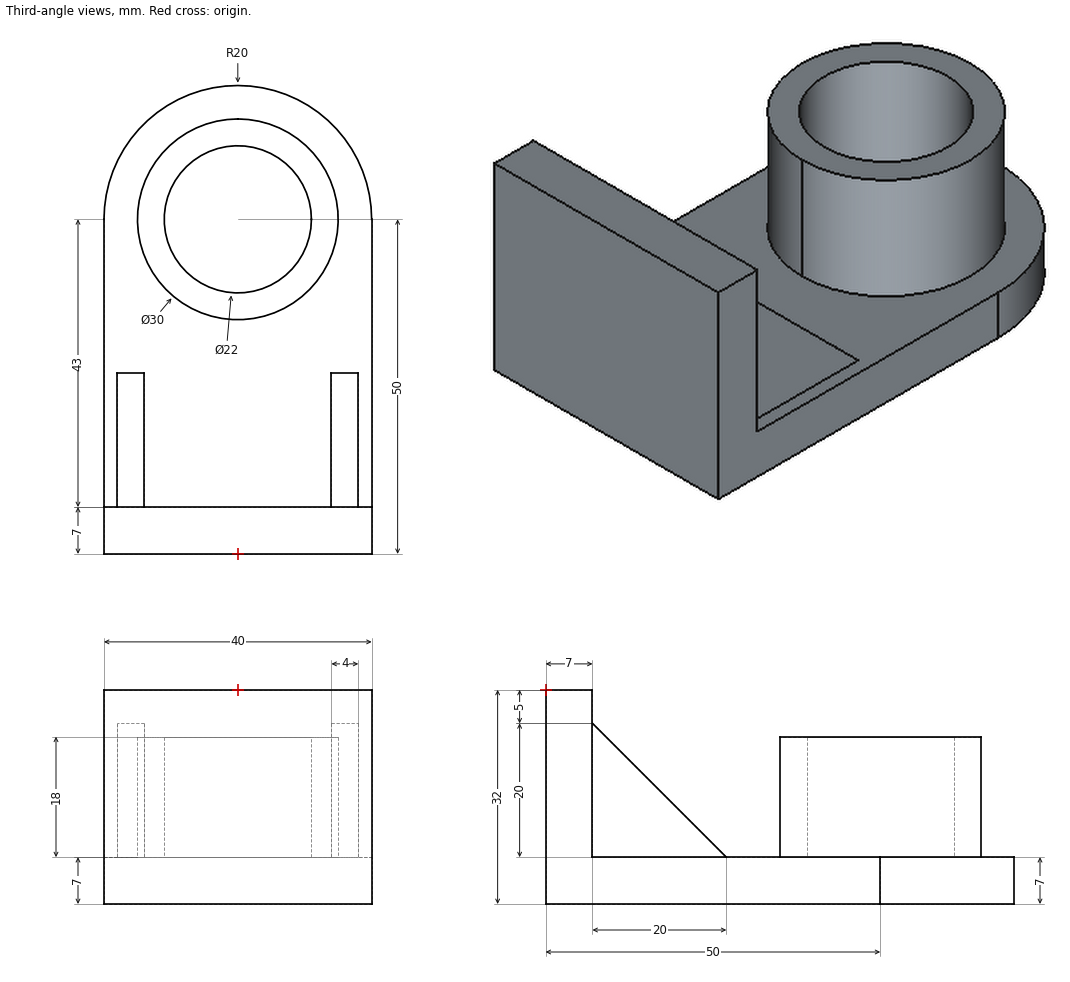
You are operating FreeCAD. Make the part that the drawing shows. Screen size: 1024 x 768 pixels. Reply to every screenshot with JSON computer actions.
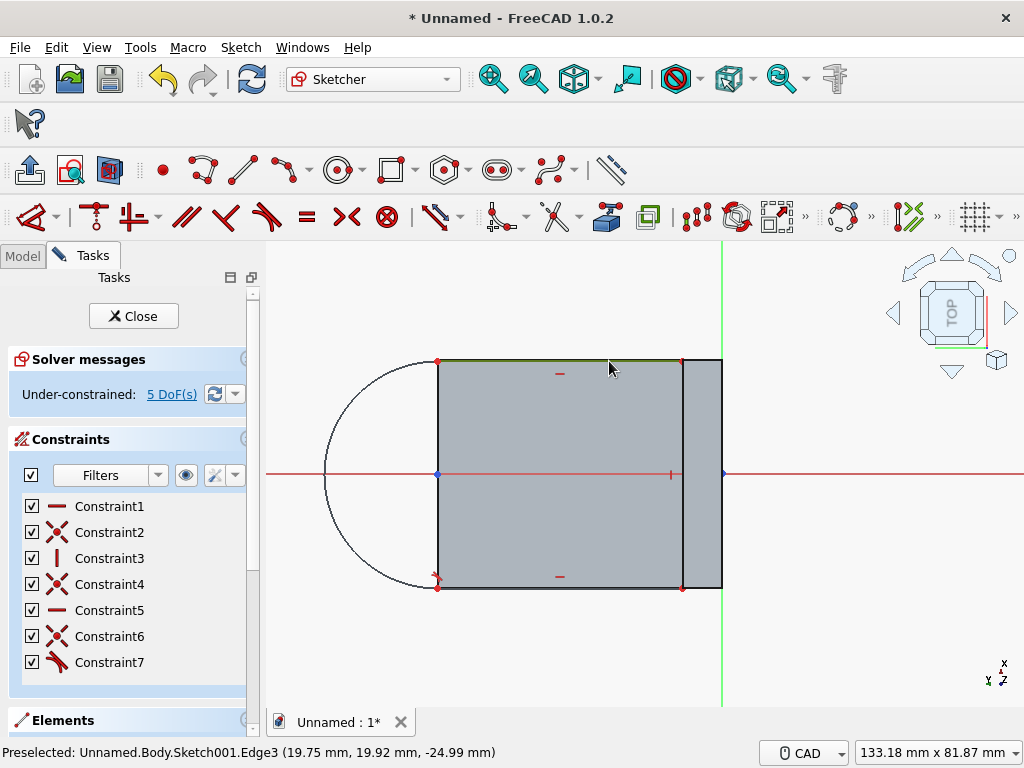
{"action": "left_click", "coordinate": [346, 408]}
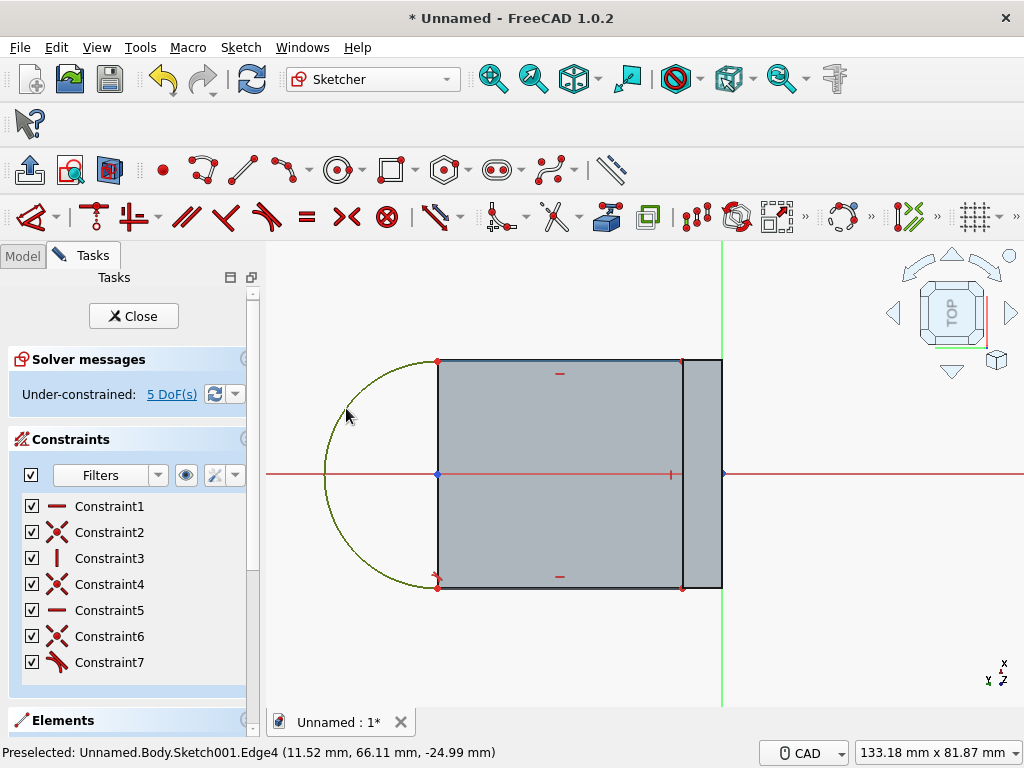
{"action": "left_click", "coordinate": [268, 218]}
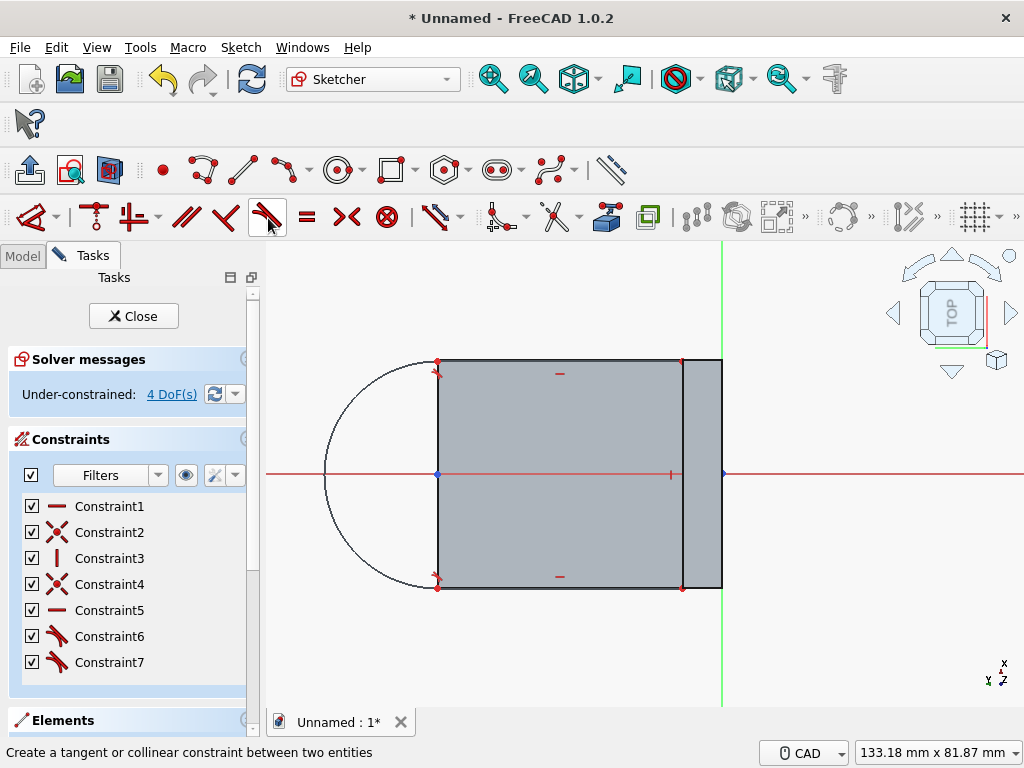
{"action": "left_click", "coordinate": [438, 475]}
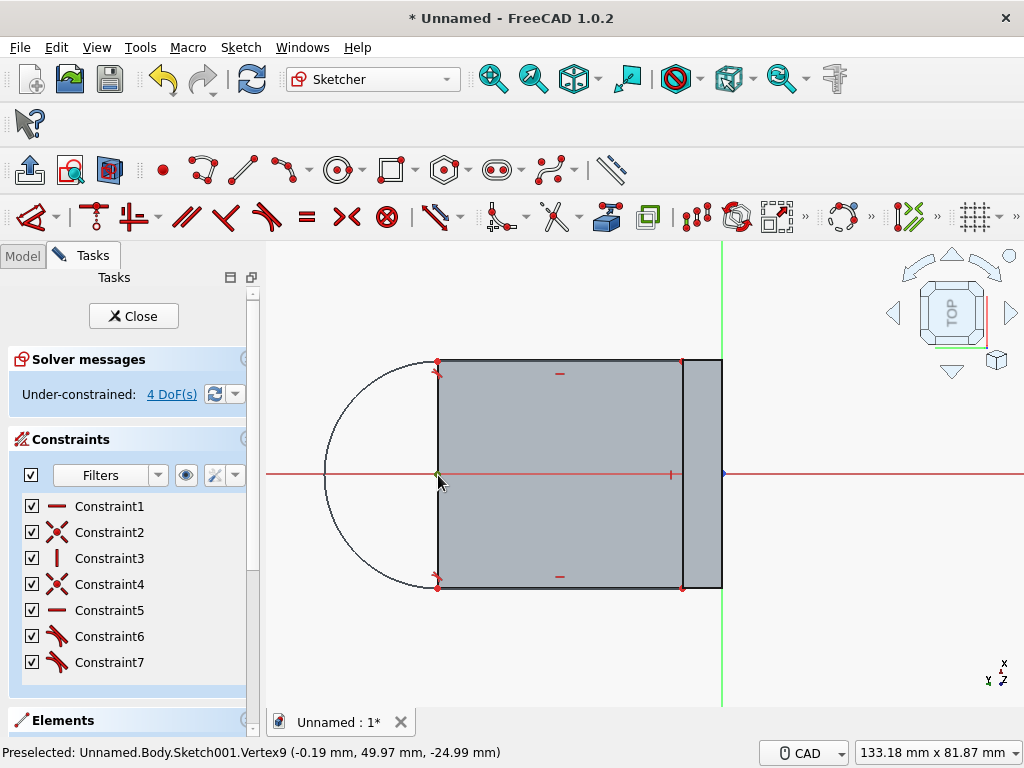
{"action": "left_click", "coordinate": [375, 474]}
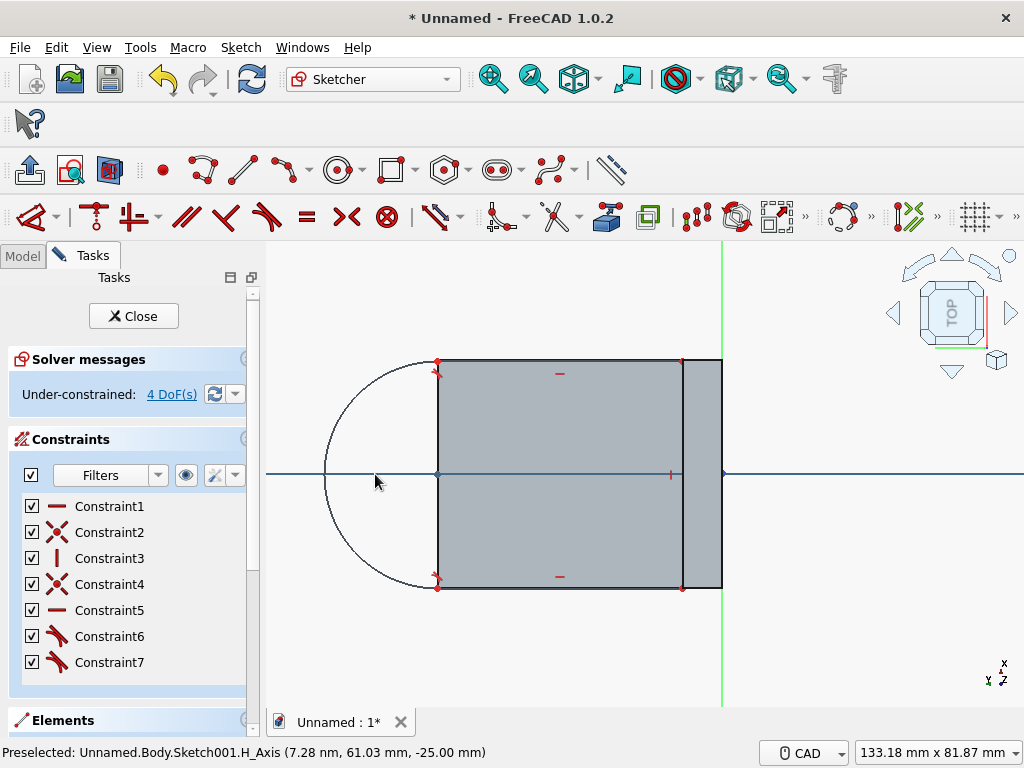
{"action": "left_click", "coordinate": [94, 218]}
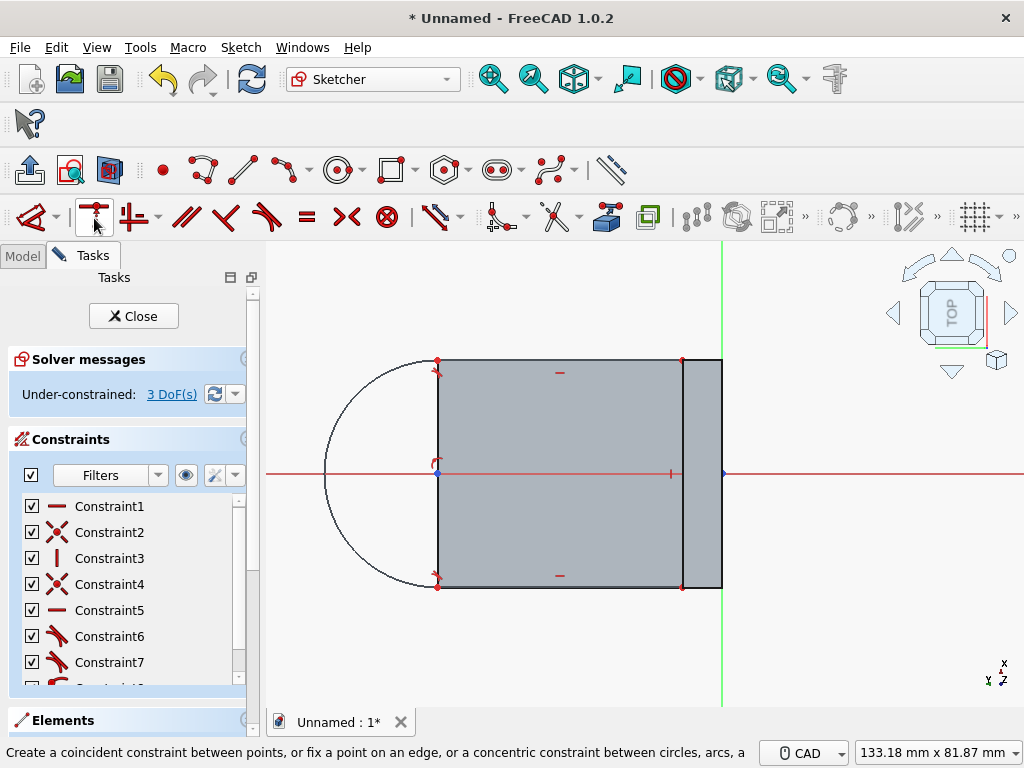
{"action": "left_click", "coordinate": [32, 218]}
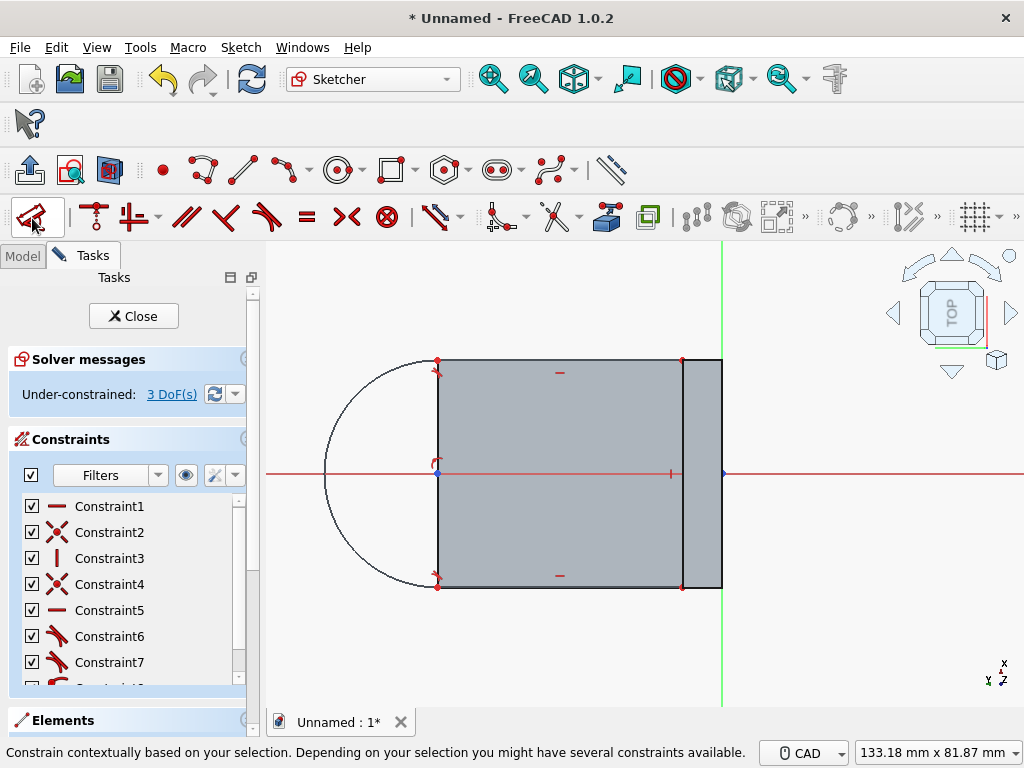
{"action": "left_click", "coordinate": [346, 407]}
{"action": "left_click", "coordinate": [320, 388]}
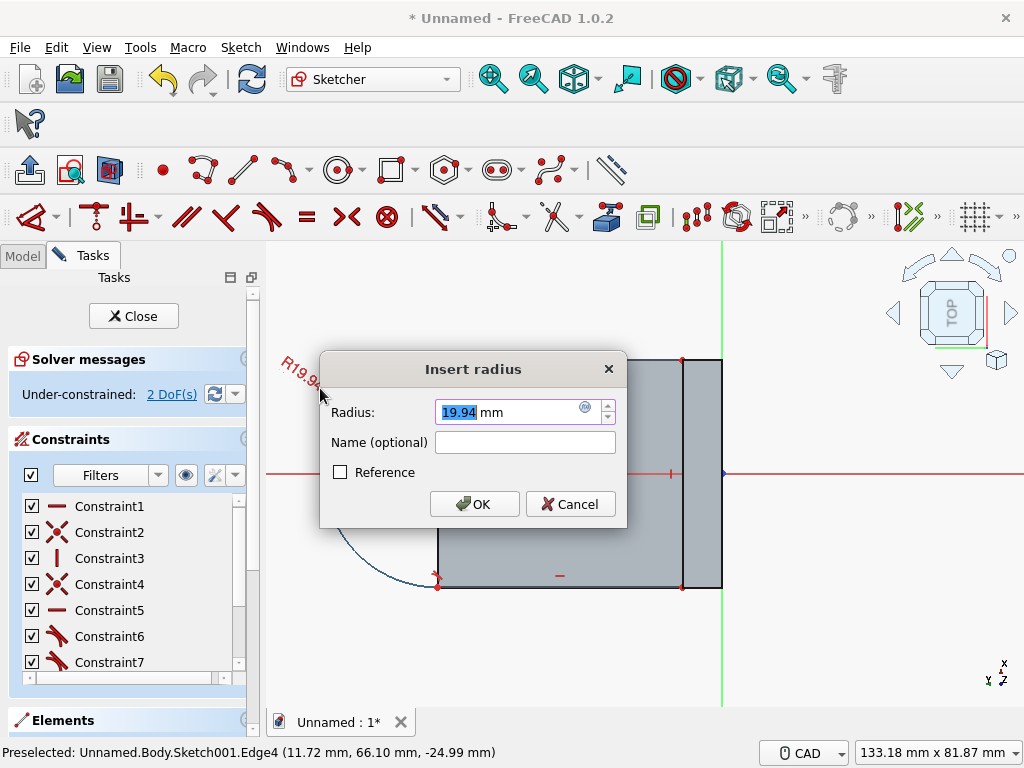
{"action": "type", "text": "20"}
{"action": "key", "text": "Return"}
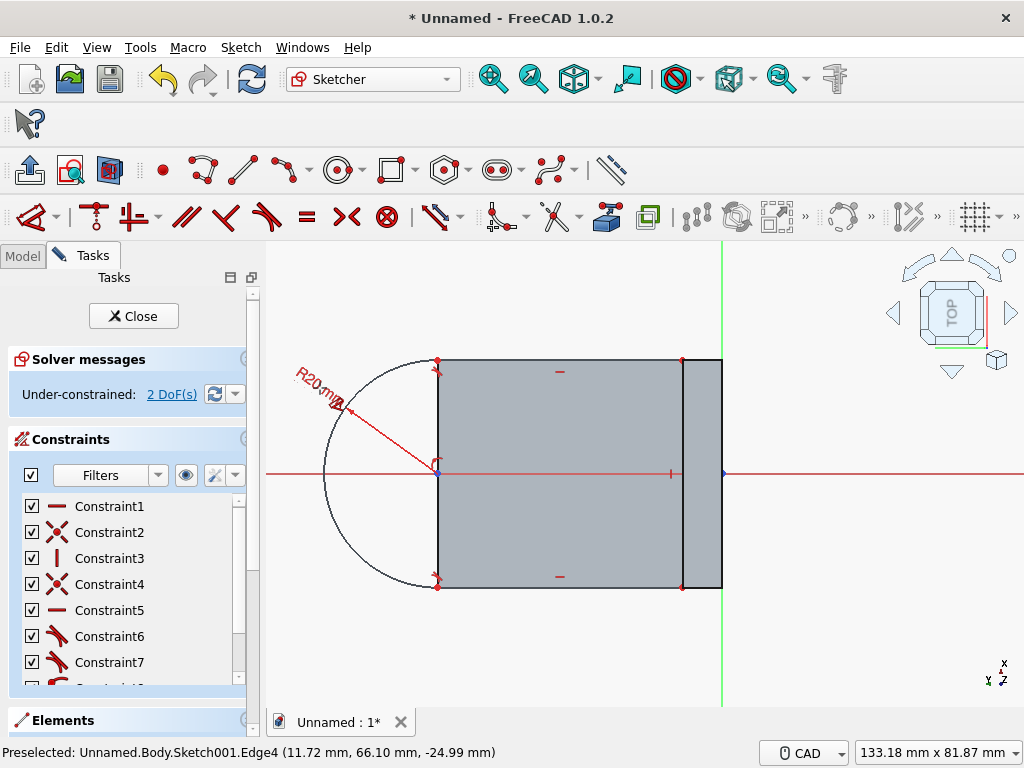
{"action": "left_click", "coordinate": [511, 588]}
{"action": "left_click", "coordinate": [560, 622]}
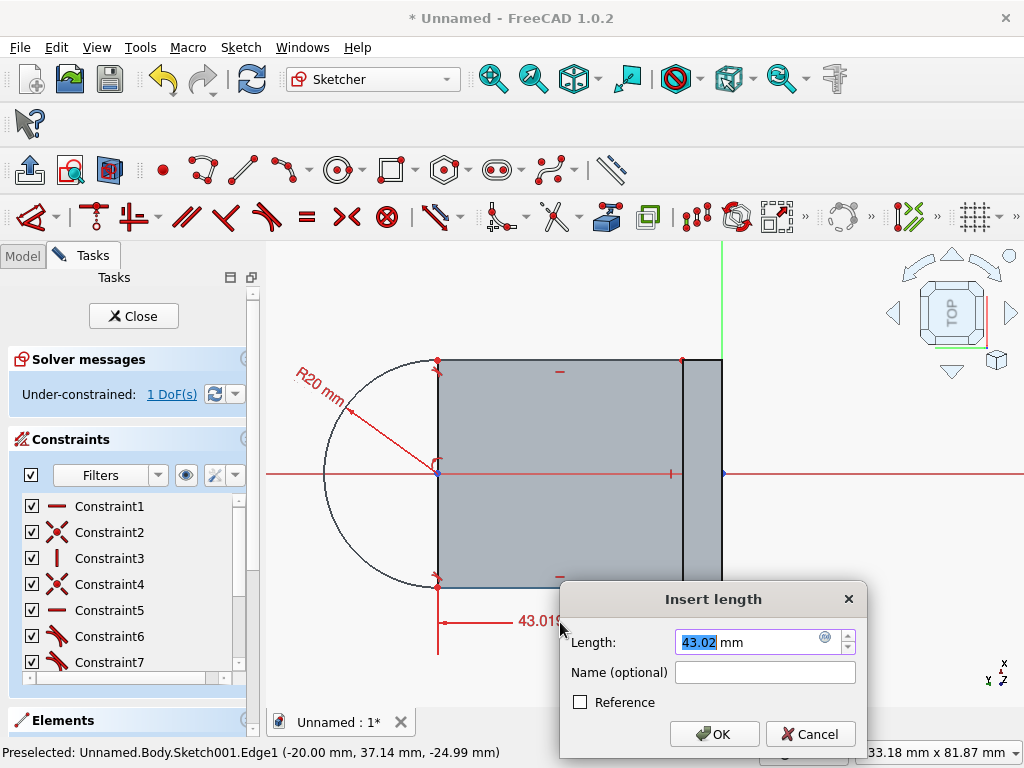
{"action": "type", "text": "43"}
{"action": "key", "text": "Return"}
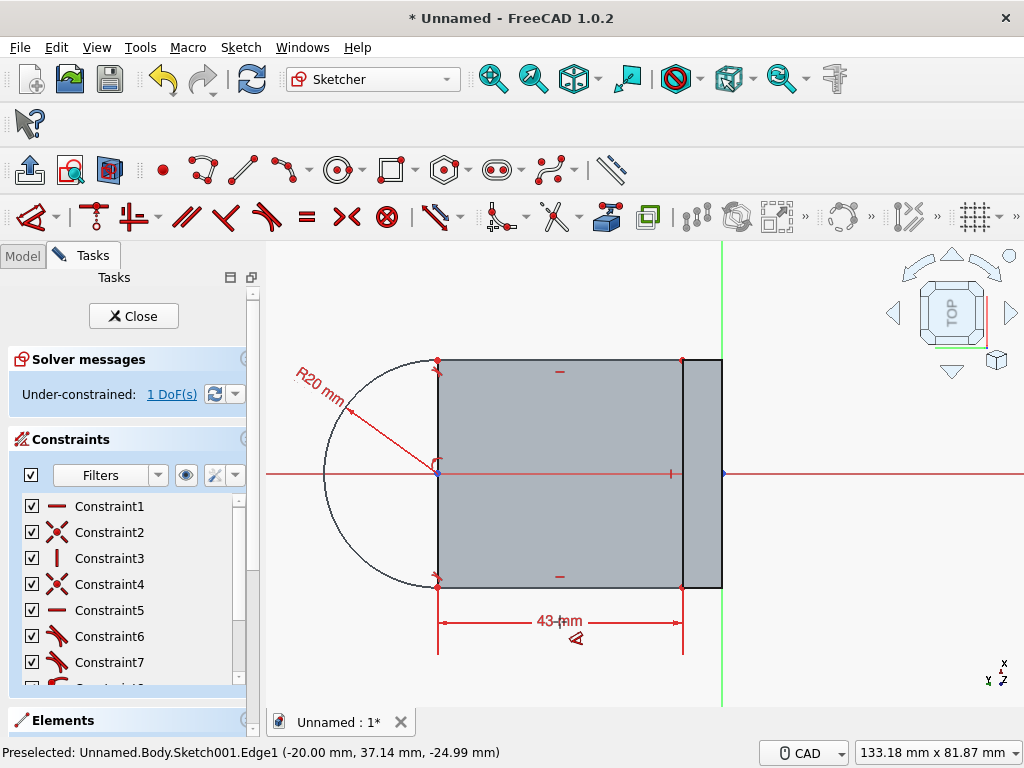
{"action": "left_click", "coordinate": [683, 588]}
{"action": "left_click", "coordinate": [703, 622]}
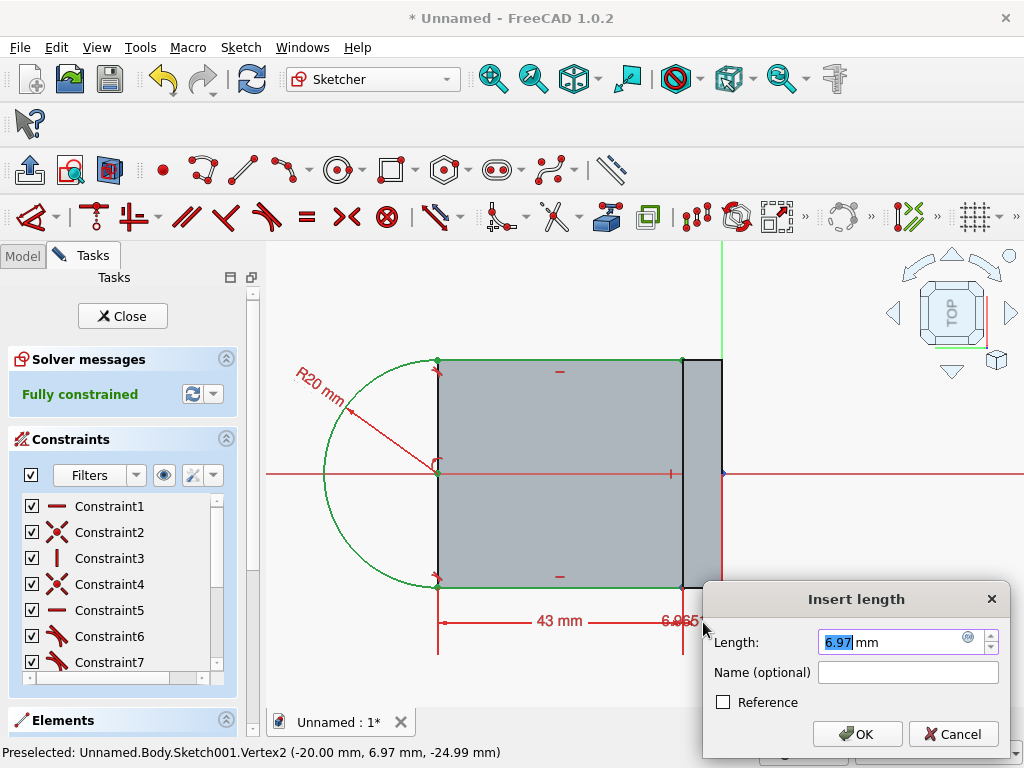
{"action": "type", "text": "7"}
{"action": "key", "text": "Return"}
{"action": "key", "text": "Escape"}